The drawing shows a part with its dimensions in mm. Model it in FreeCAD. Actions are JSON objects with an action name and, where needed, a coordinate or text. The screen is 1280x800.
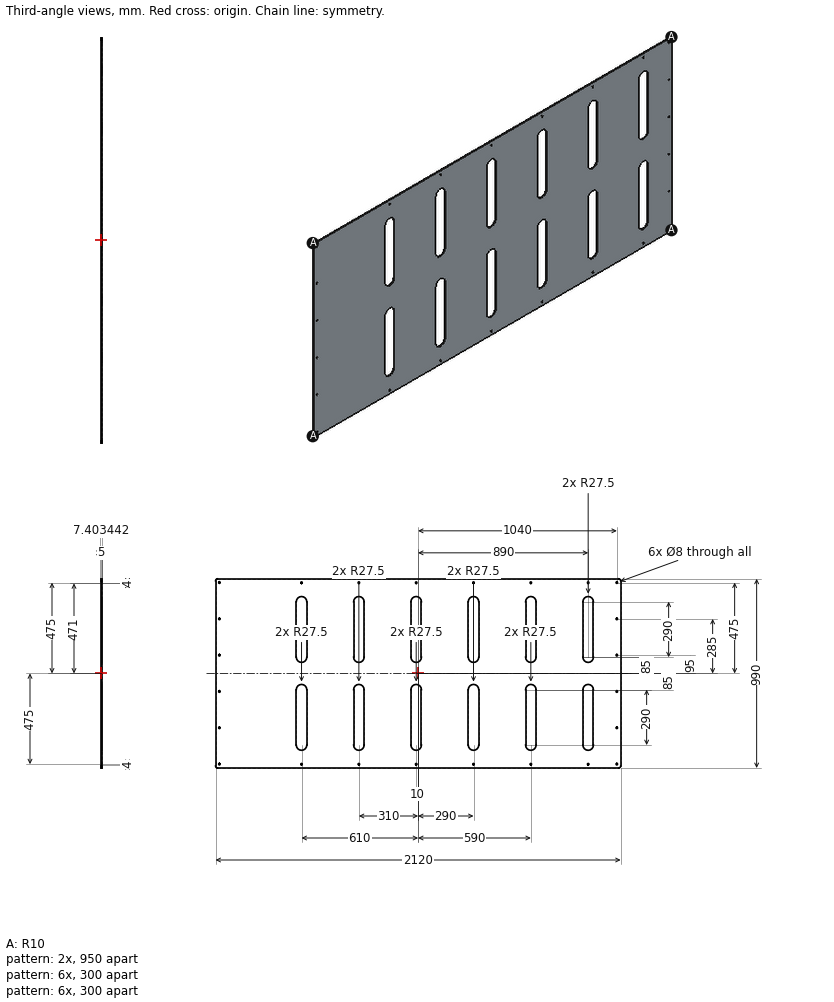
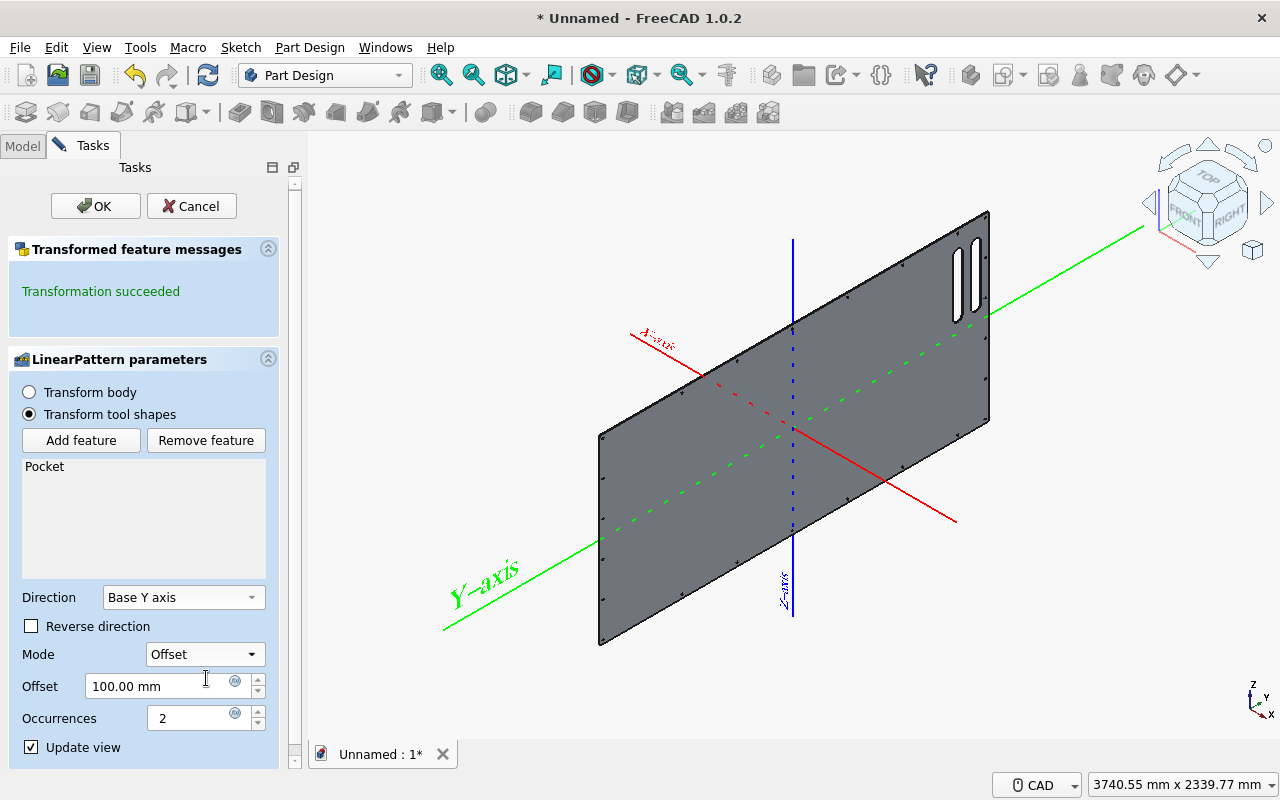
{"action": "triple_click", "coordinate": [168, 686]}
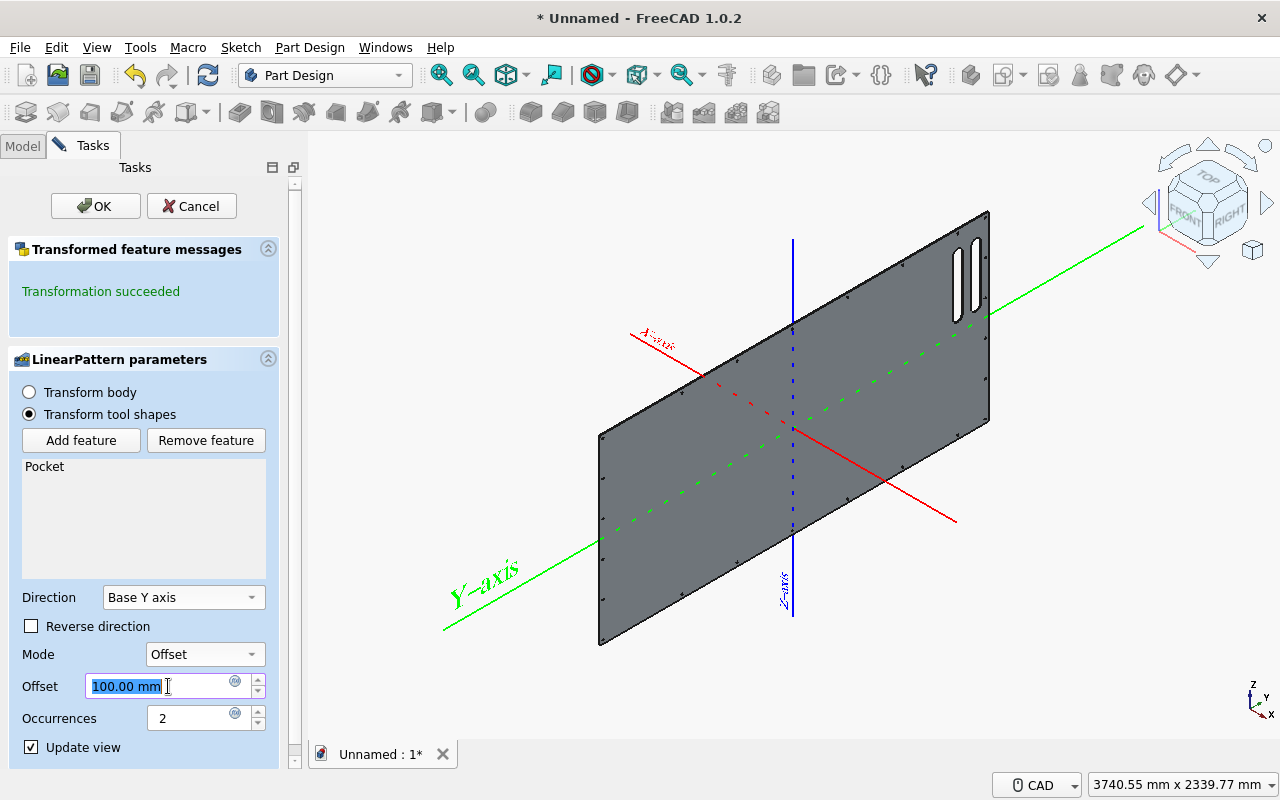
{"action": "type", "text": "300"}
{"action": "key", "text": "Tab"}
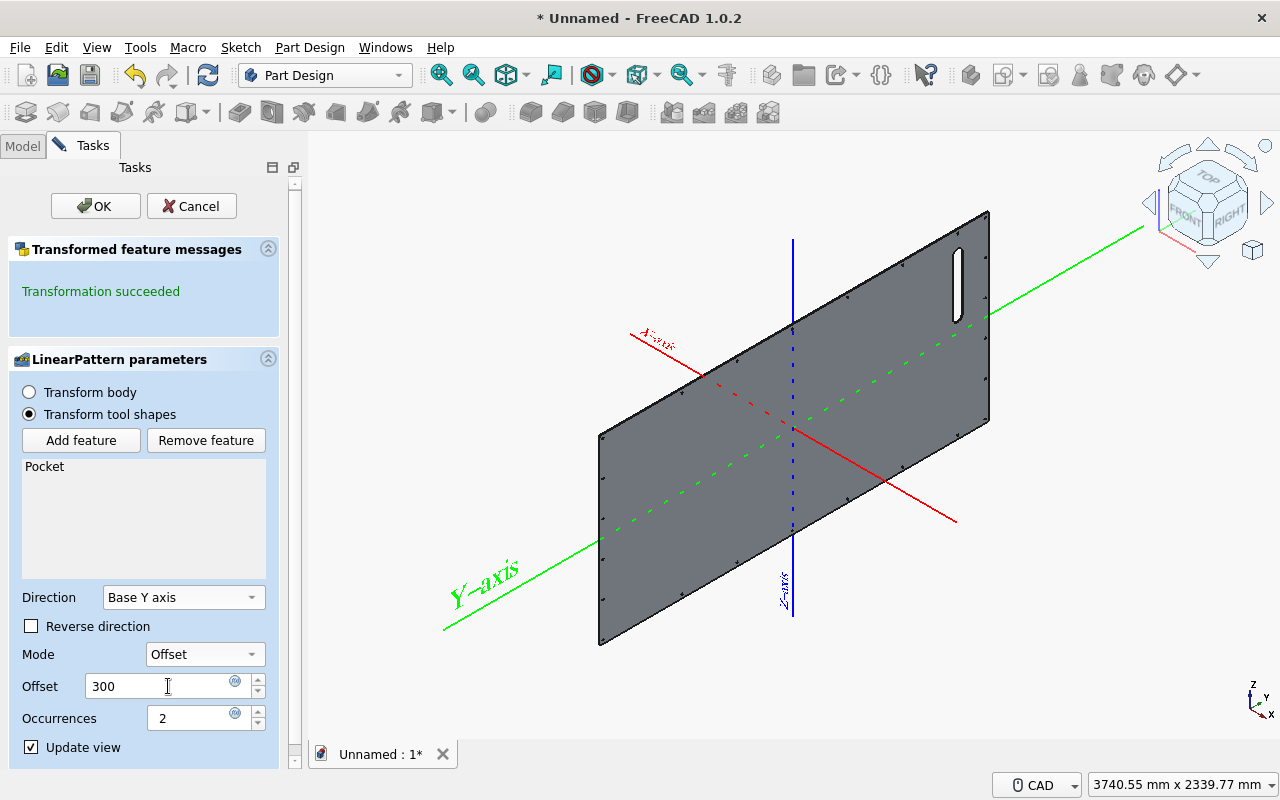
{"action": "triple_click", "coordinate": [198, 718]}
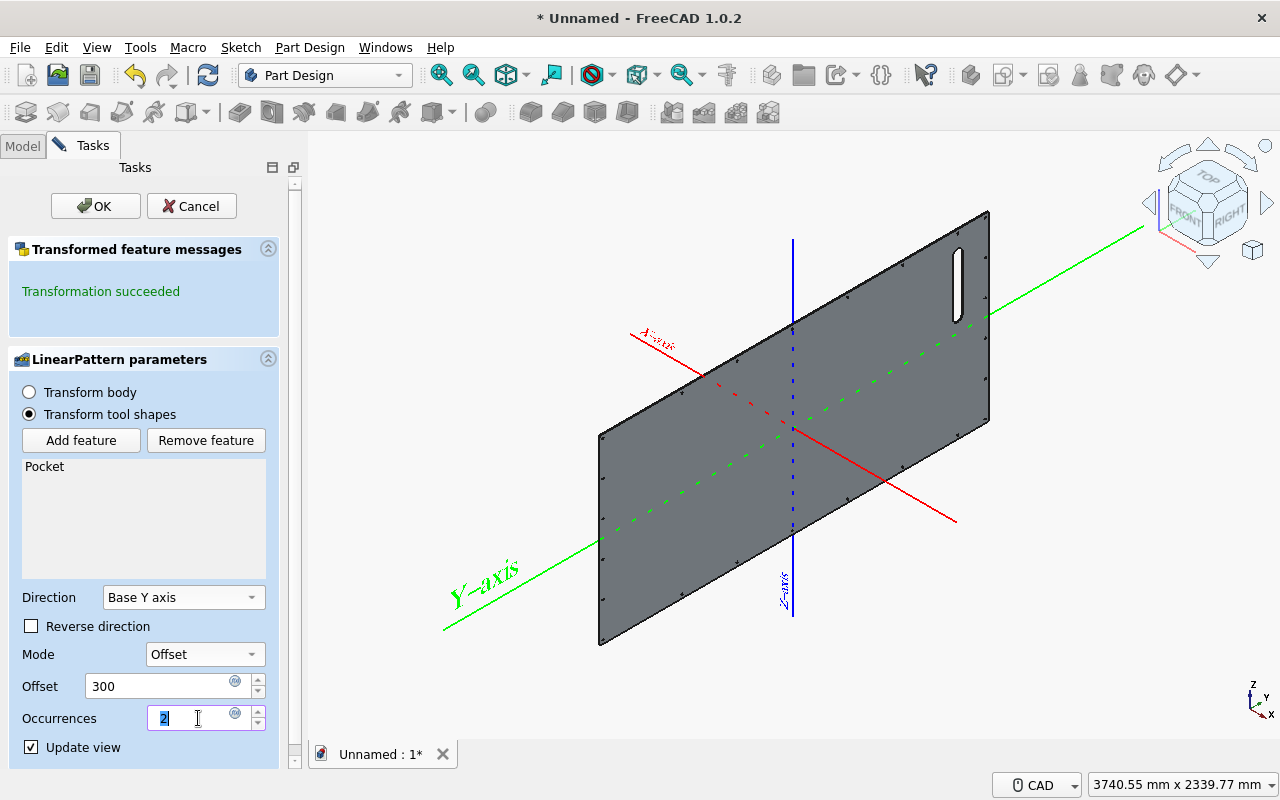
{"action": "type", "text": "6"}
{"action": "key", "text": "Tab"}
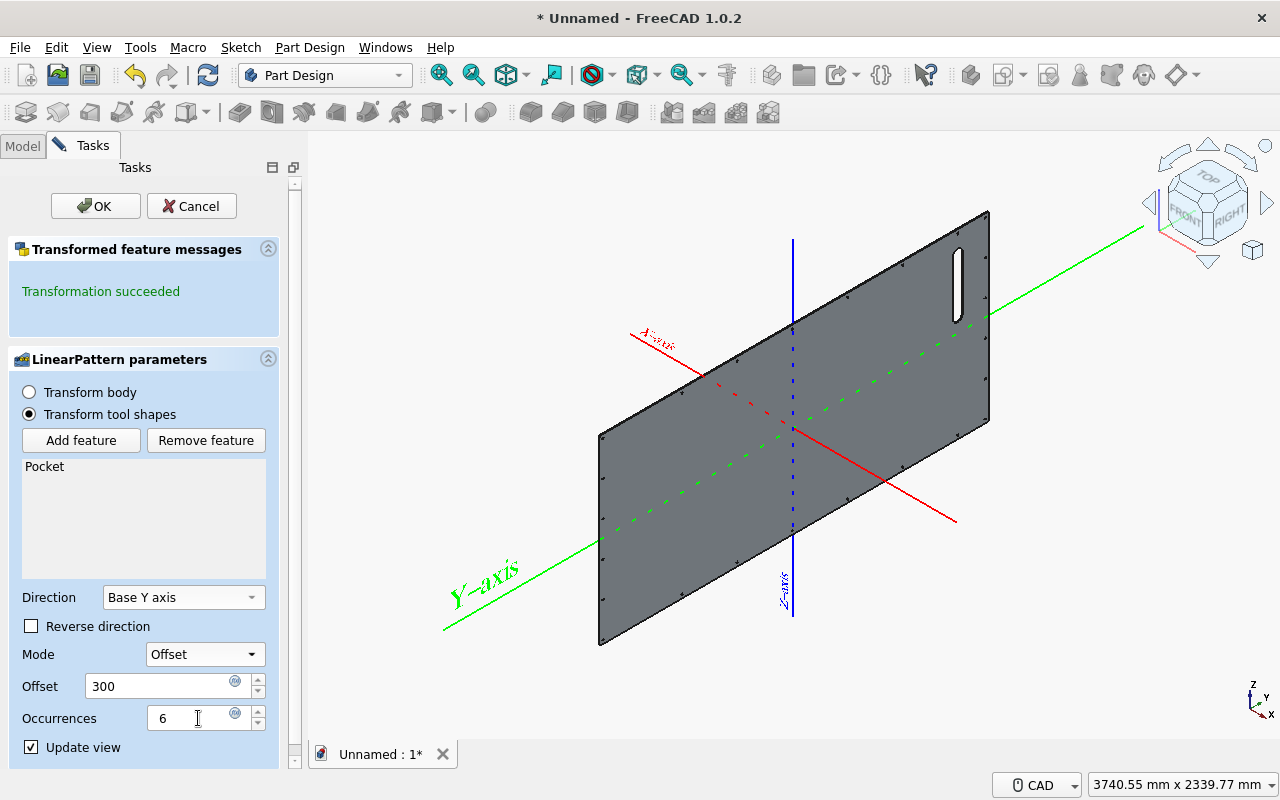
{"action": "left_click", "coordinate": [30, 626]}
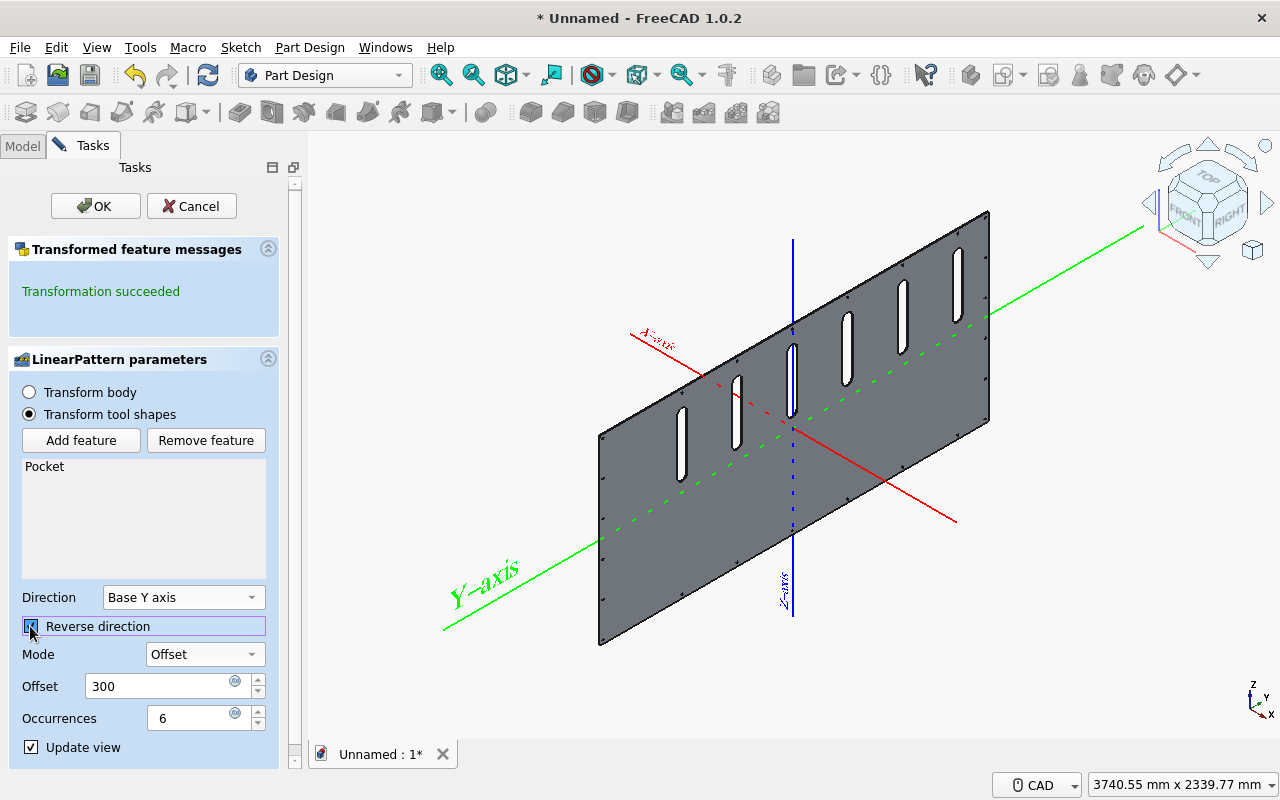
{"action": "left_click", "coordinate": [96, 206]}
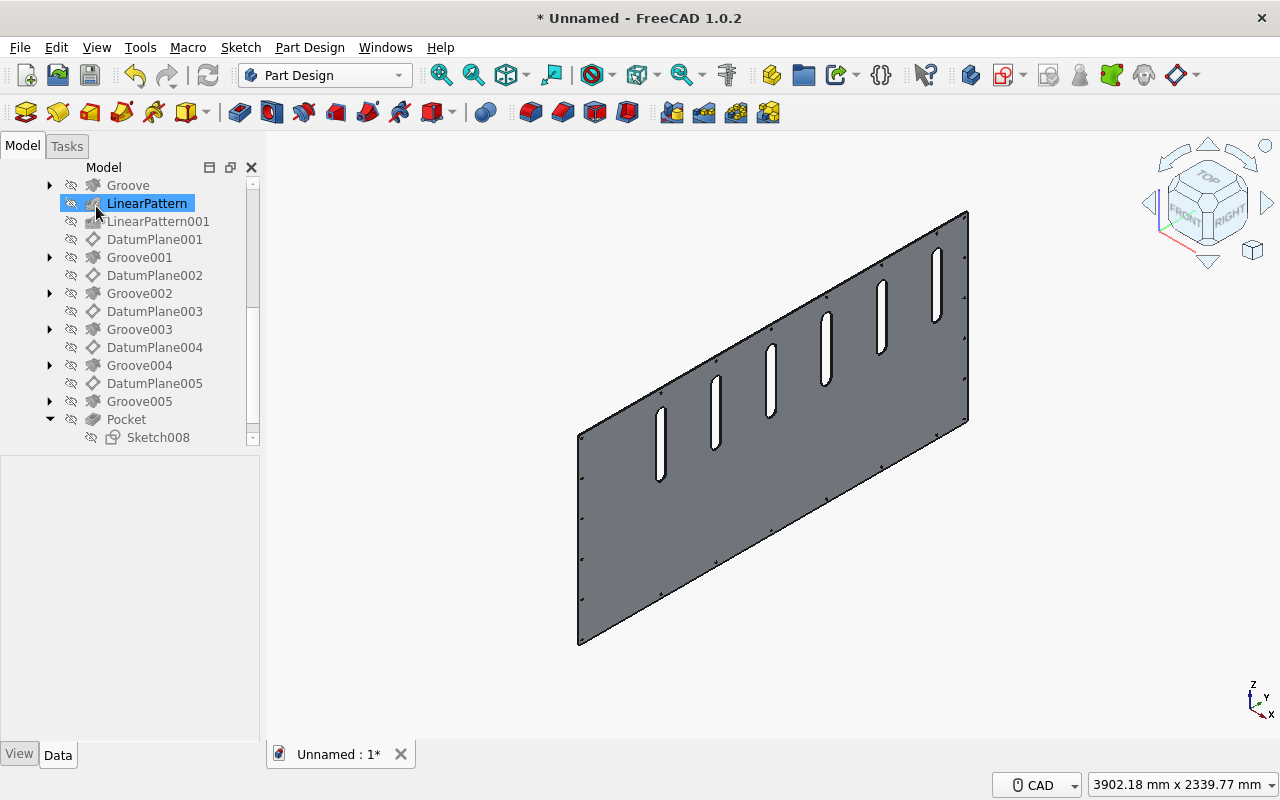
{"action": "left_click", "coordinate": [116, 419]}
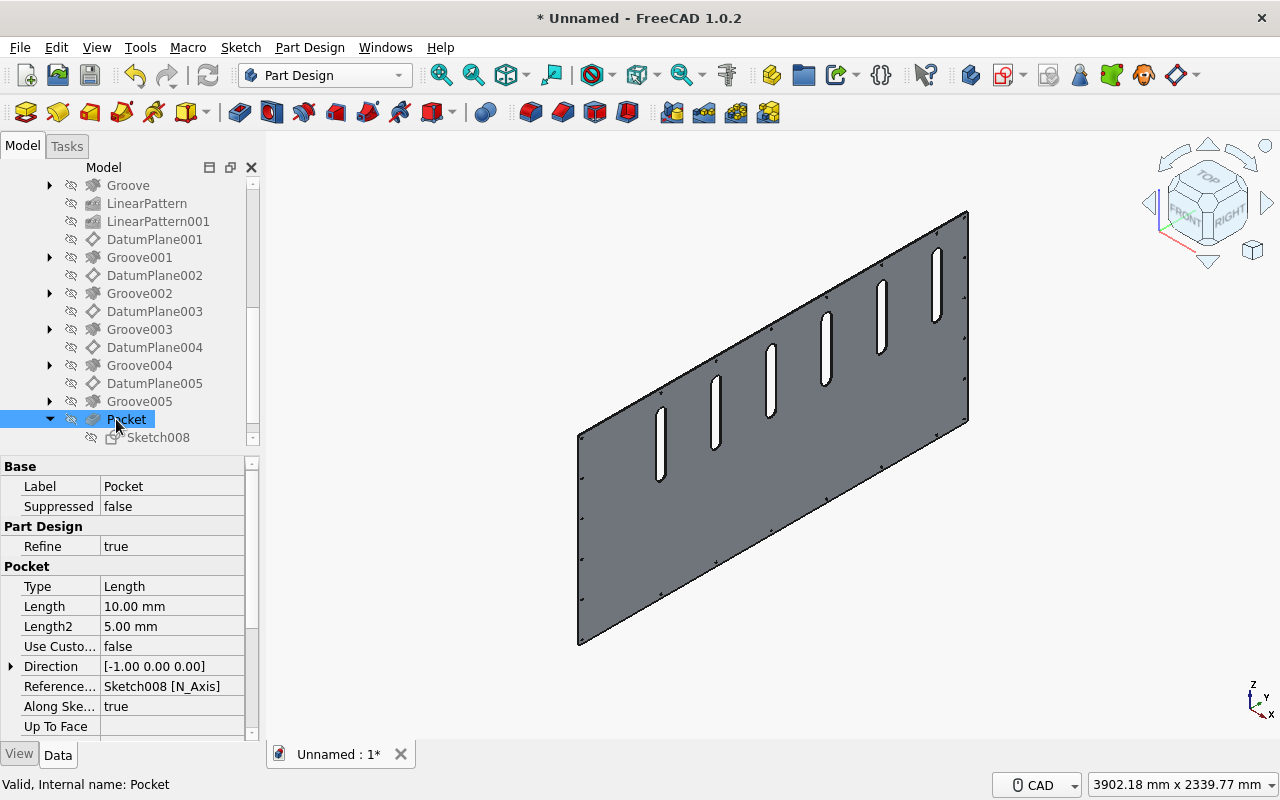
{"action": "left_click", "coordinate": [672, 112]}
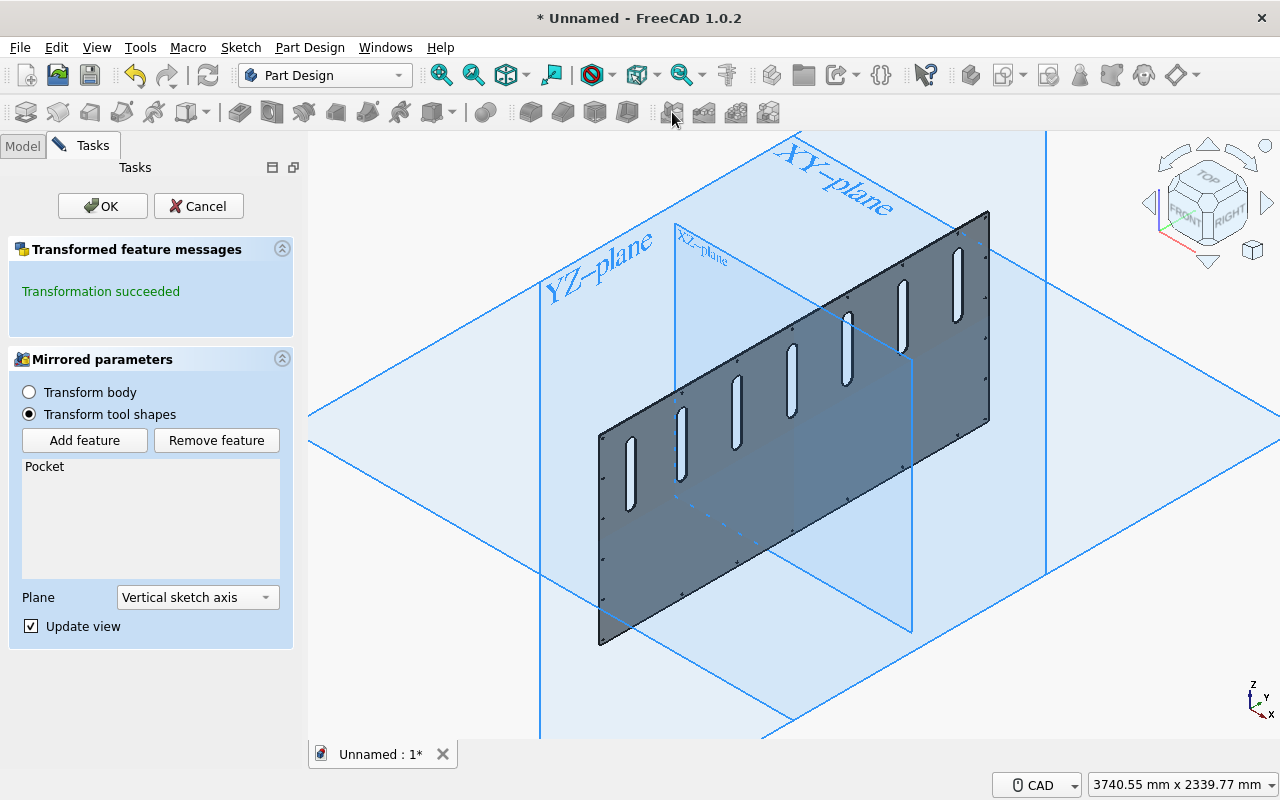
{"action": "left_click", "coordinate": [198, 598]}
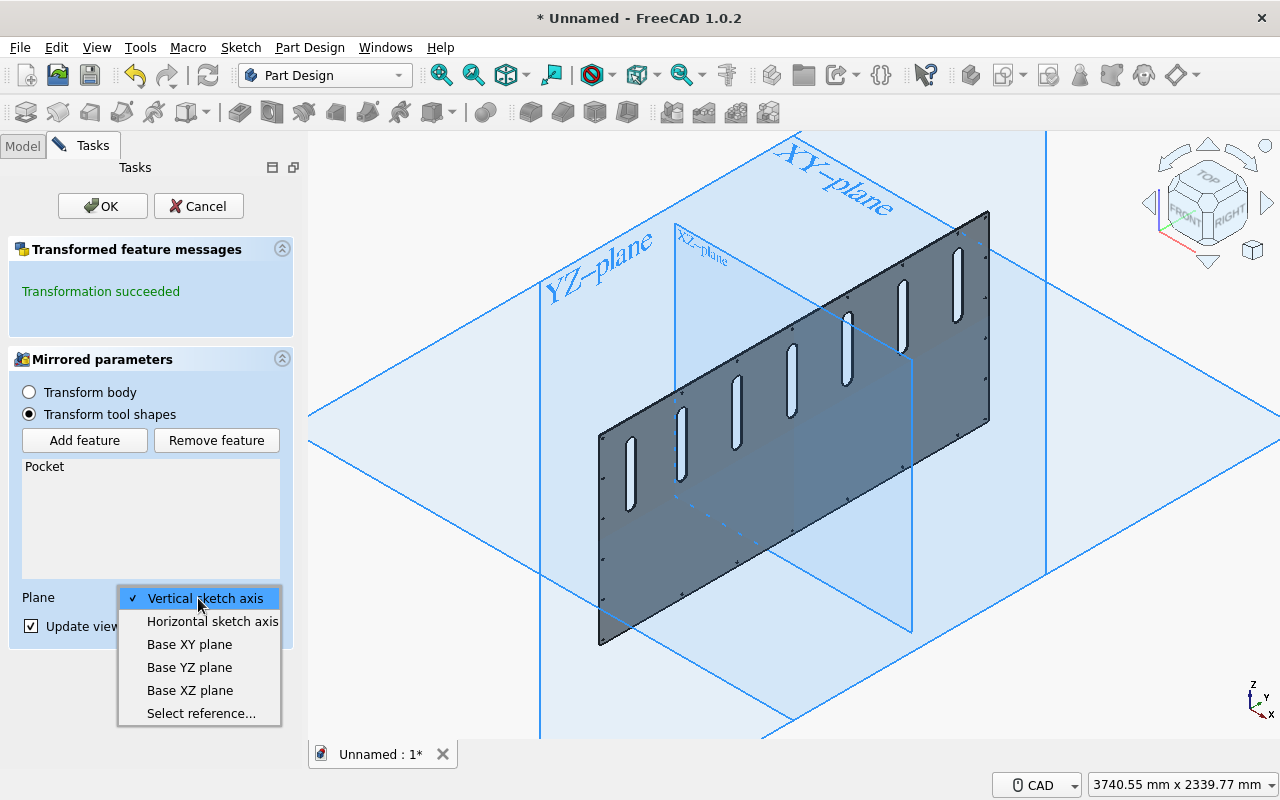
{"action": "left_click", "coordinate": [198, 644]}